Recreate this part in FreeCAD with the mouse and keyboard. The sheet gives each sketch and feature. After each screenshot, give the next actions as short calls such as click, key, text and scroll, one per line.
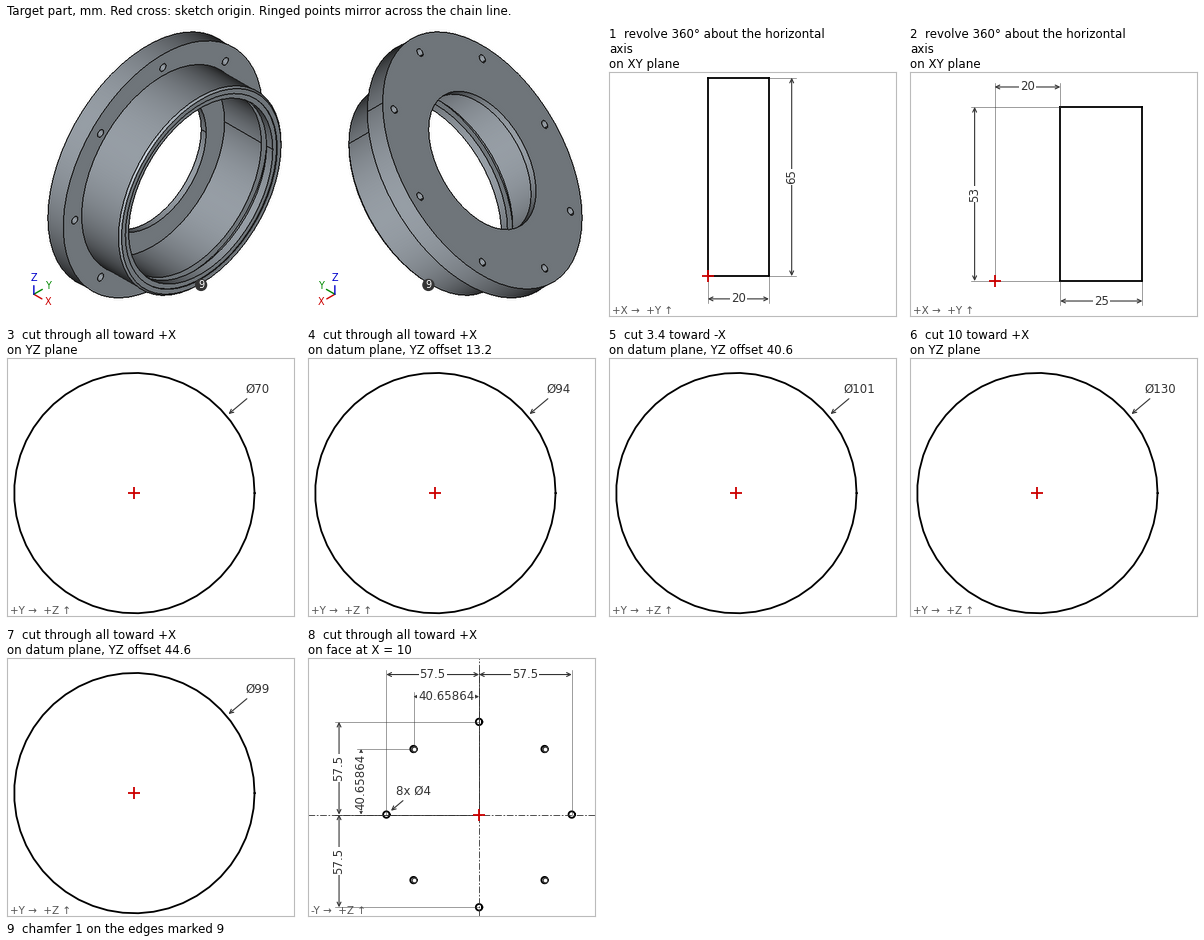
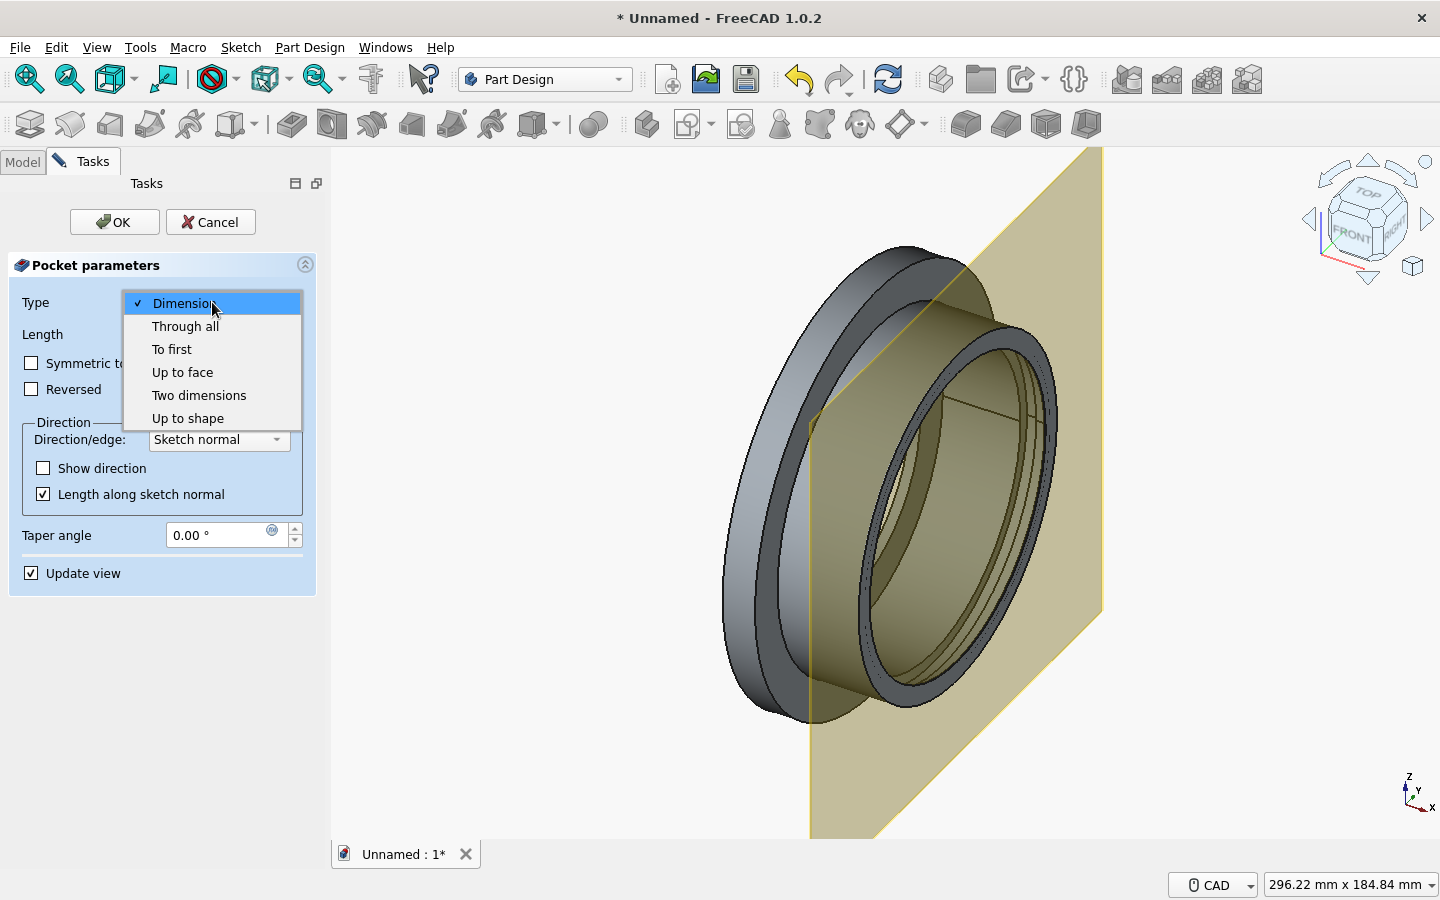
click(212, 326)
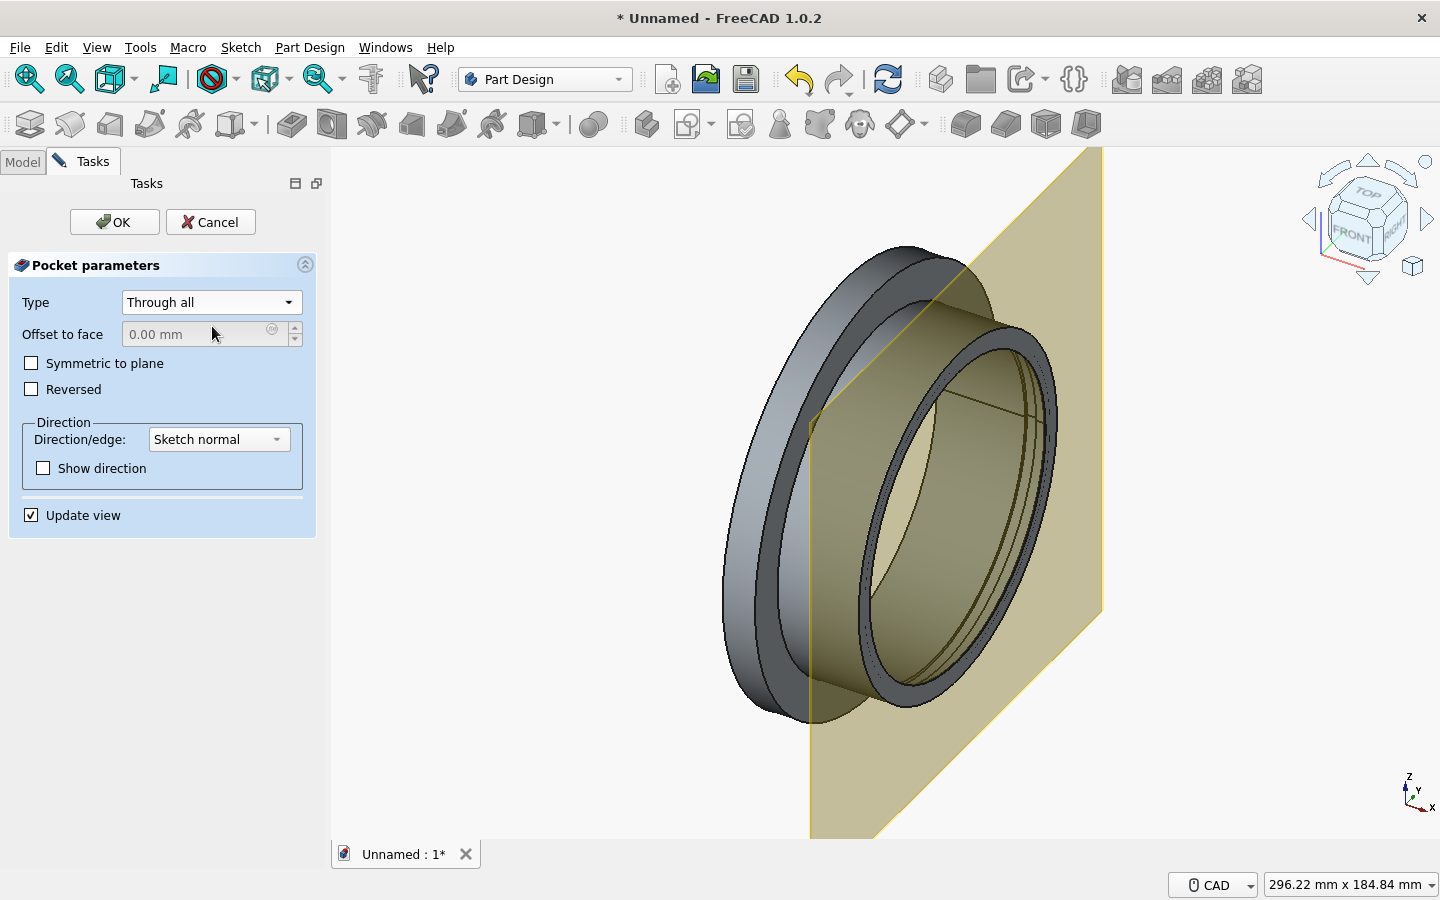
click(30, 389)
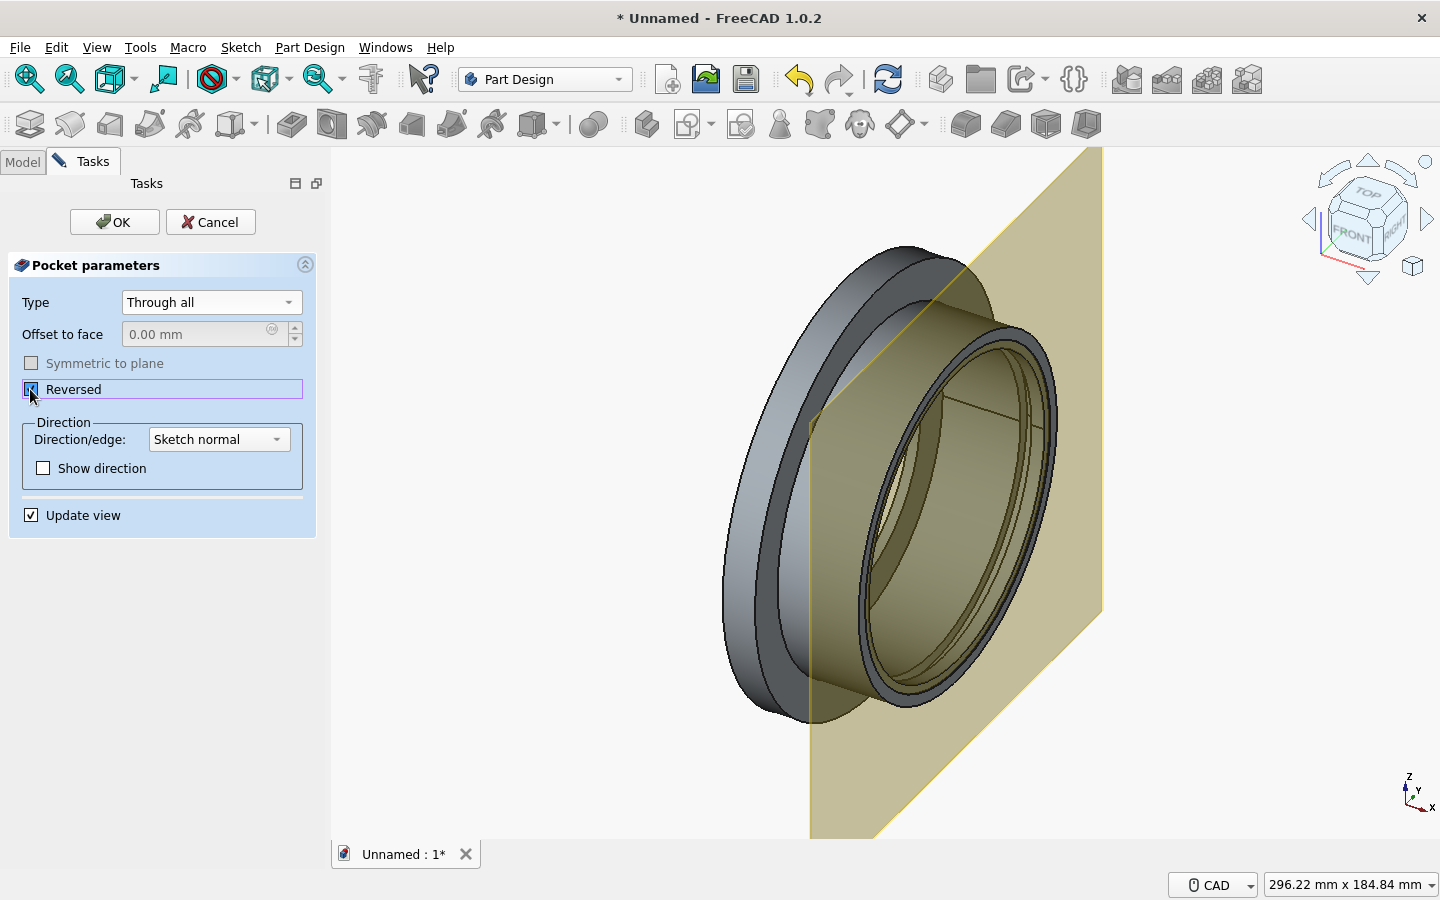
click(115, 222)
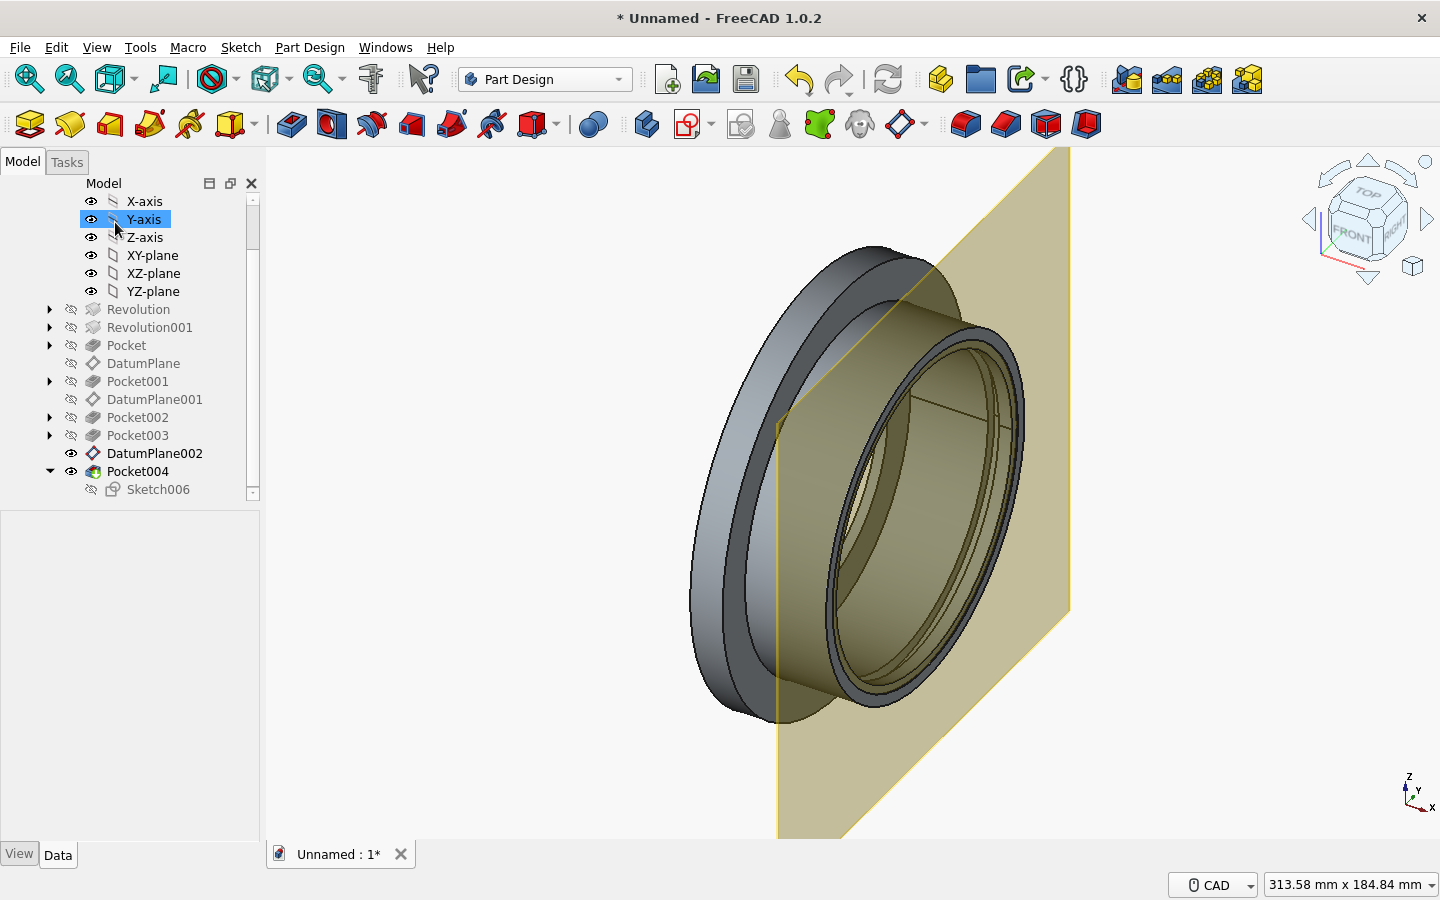
click(116, 453)
key(space)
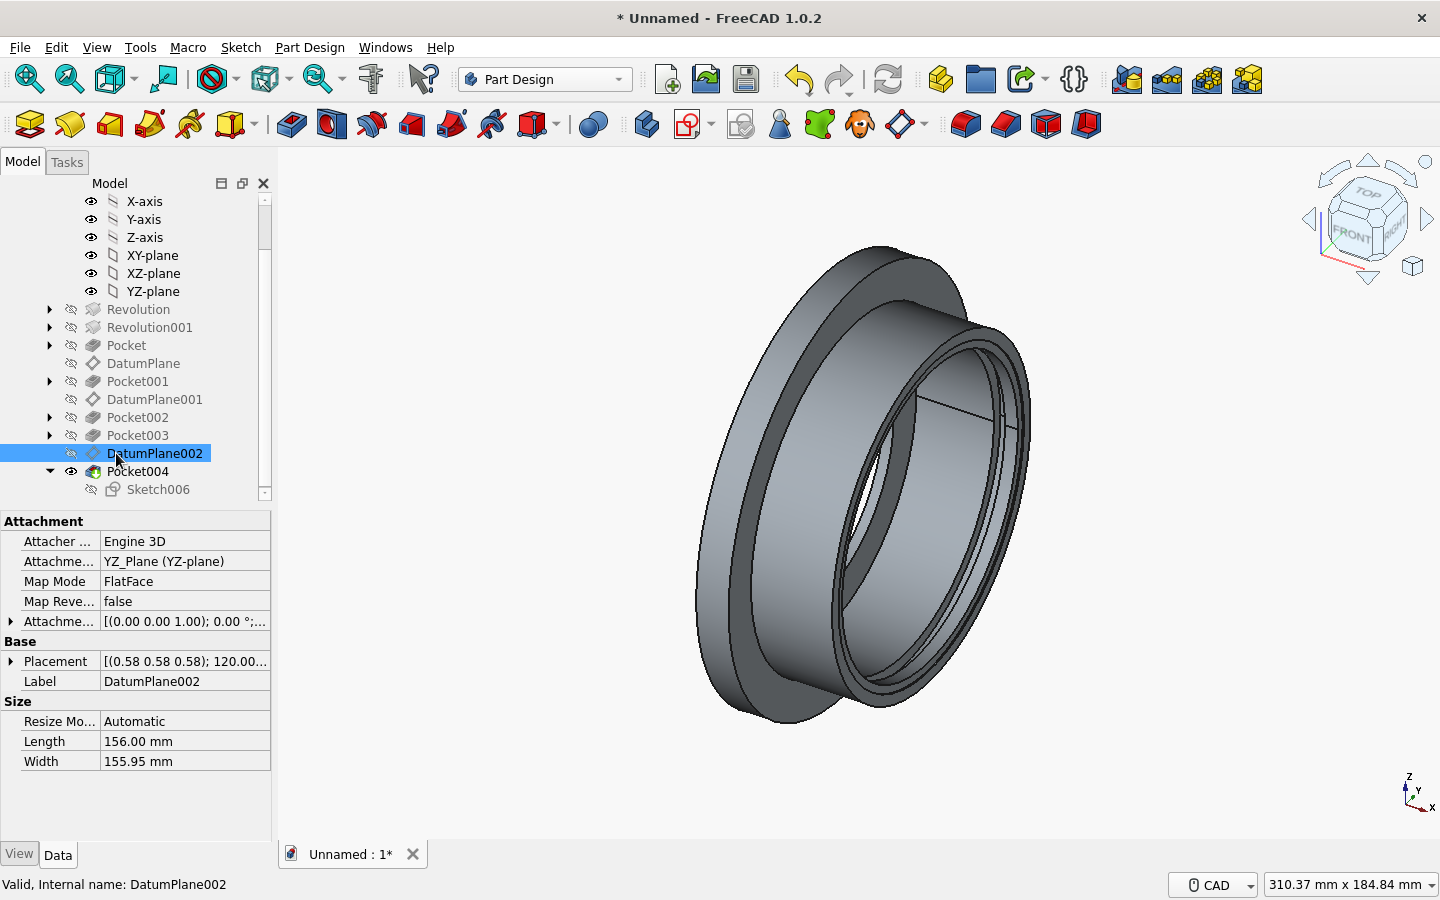
key(6)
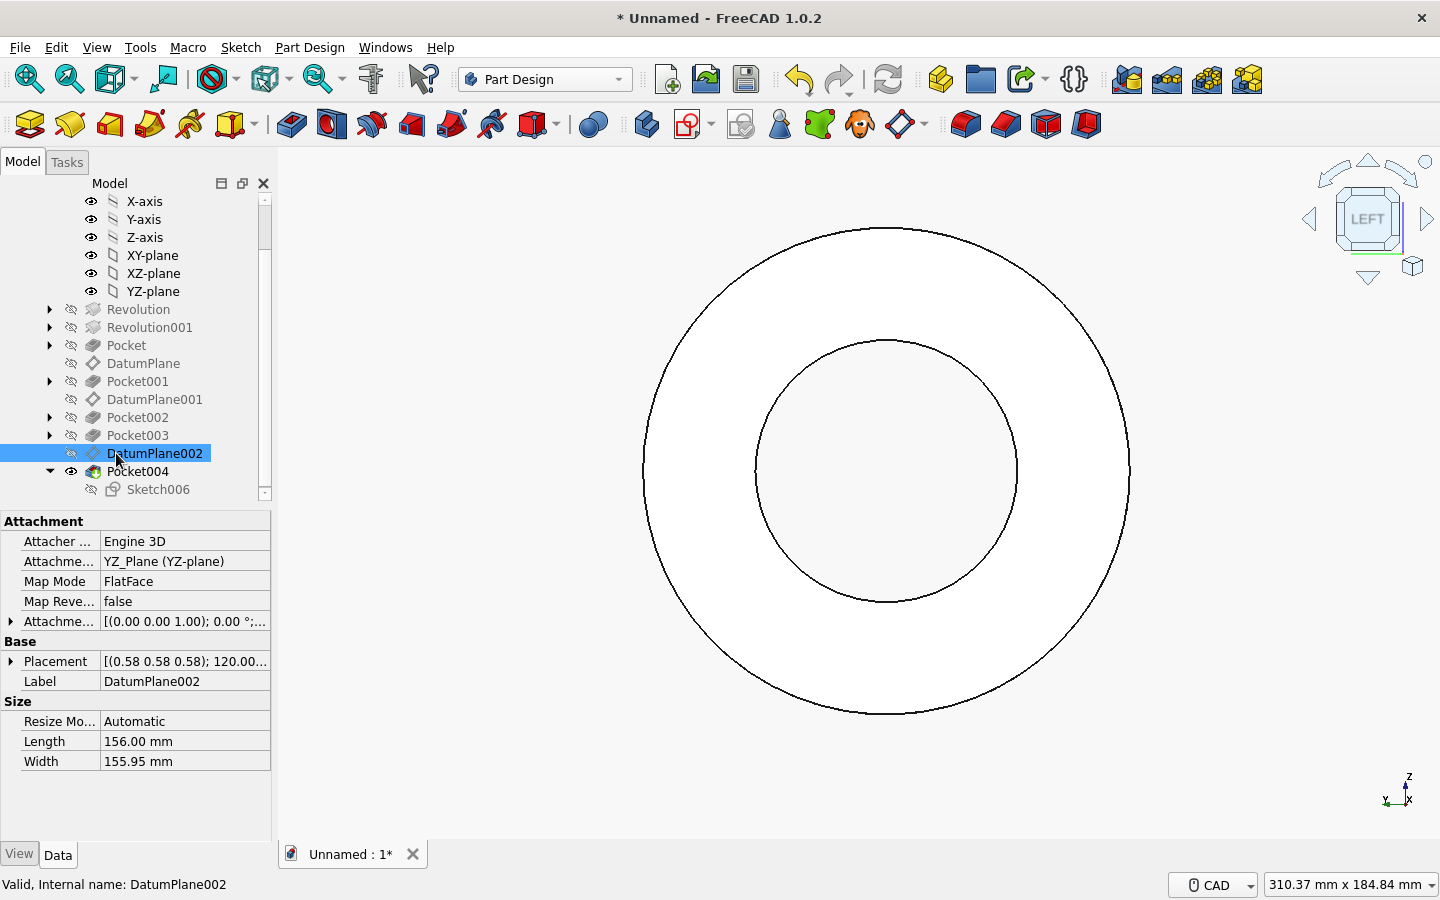
click(747, 331)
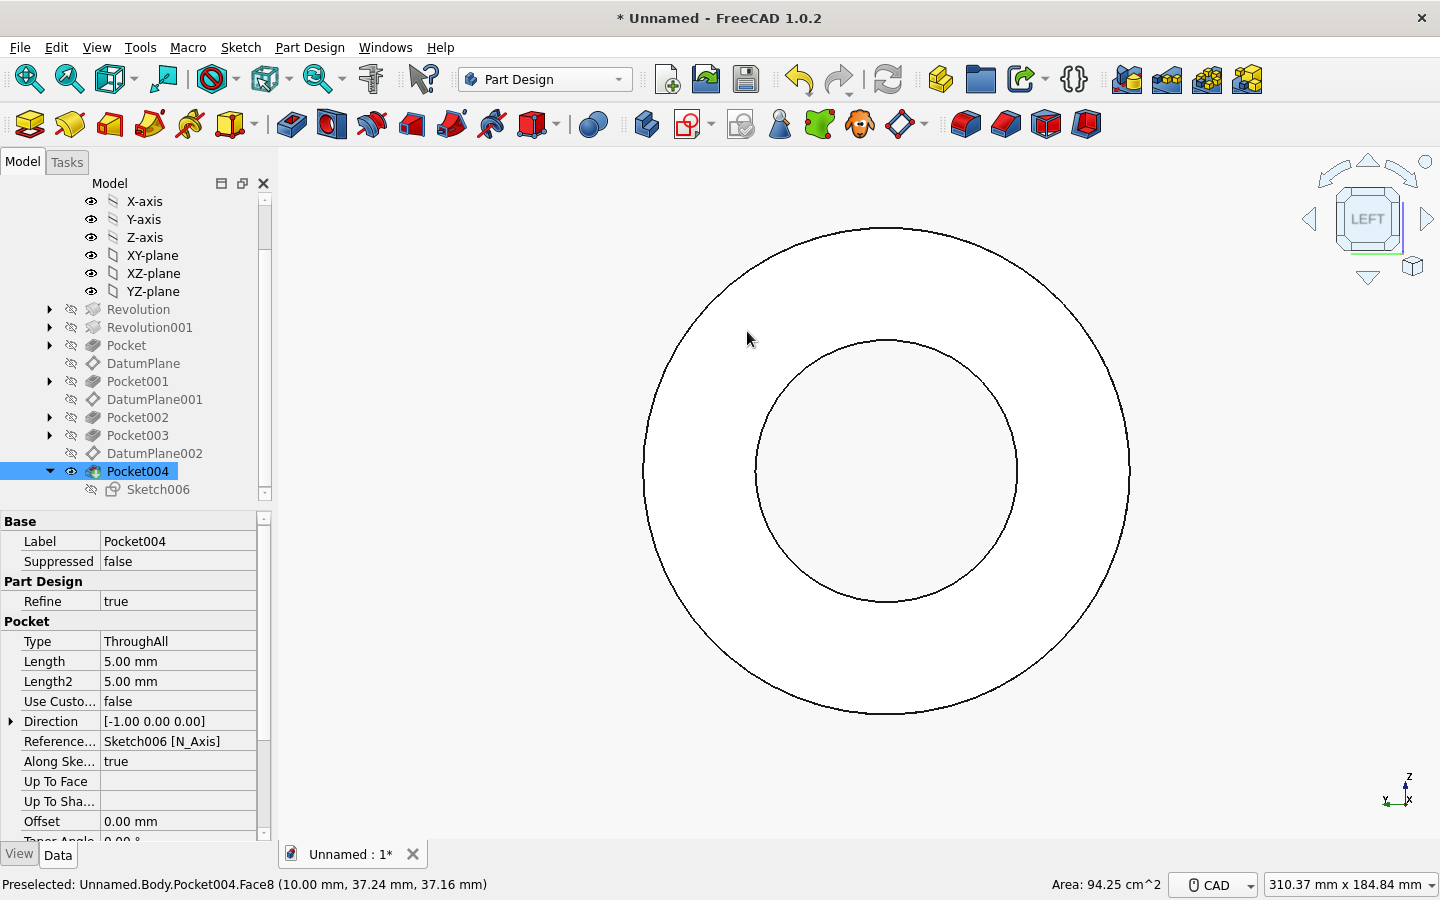
click(688, 124)